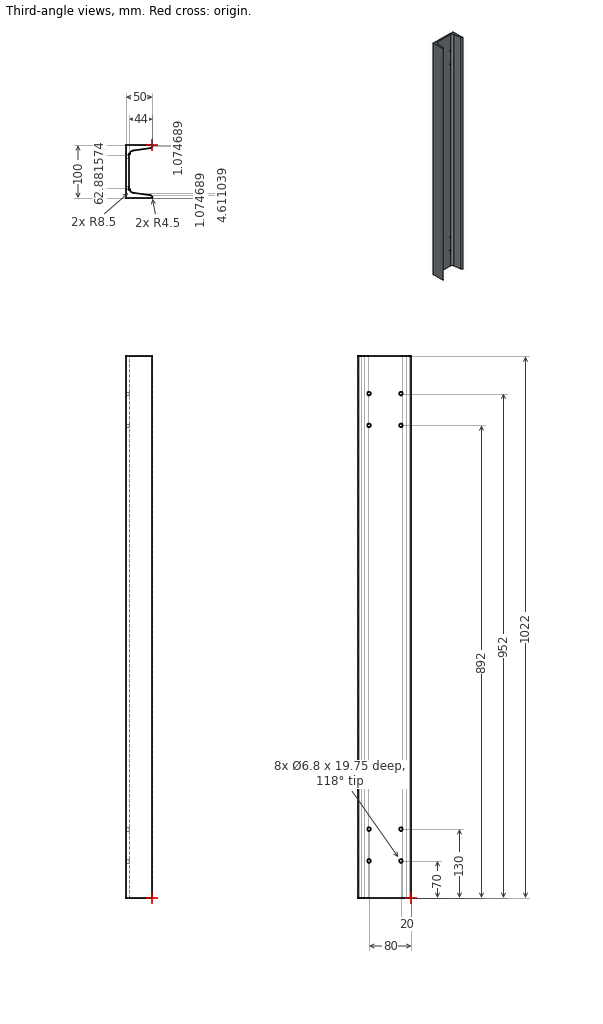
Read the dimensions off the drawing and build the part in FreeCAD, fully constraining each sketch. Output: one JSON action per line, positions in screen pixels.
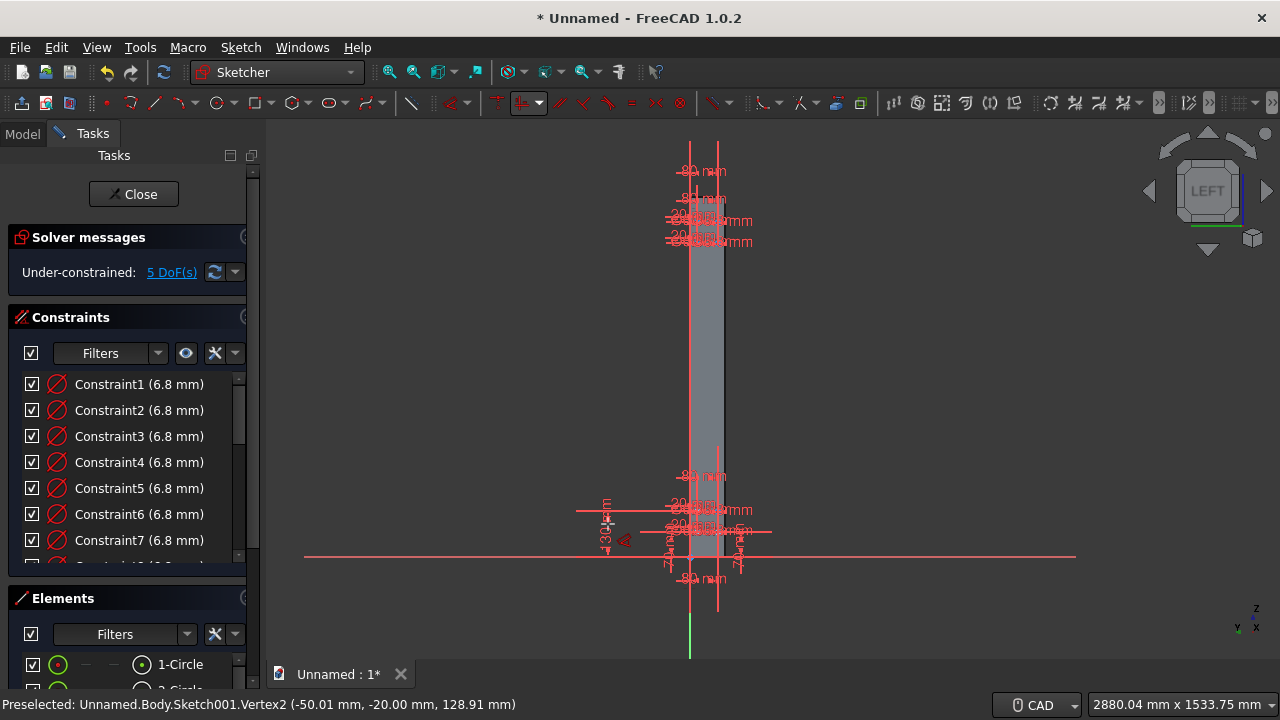
{"action": "left_click", "coordinate": [718, 512]}
{"action": "left_click", "coordinate": [776, 524]}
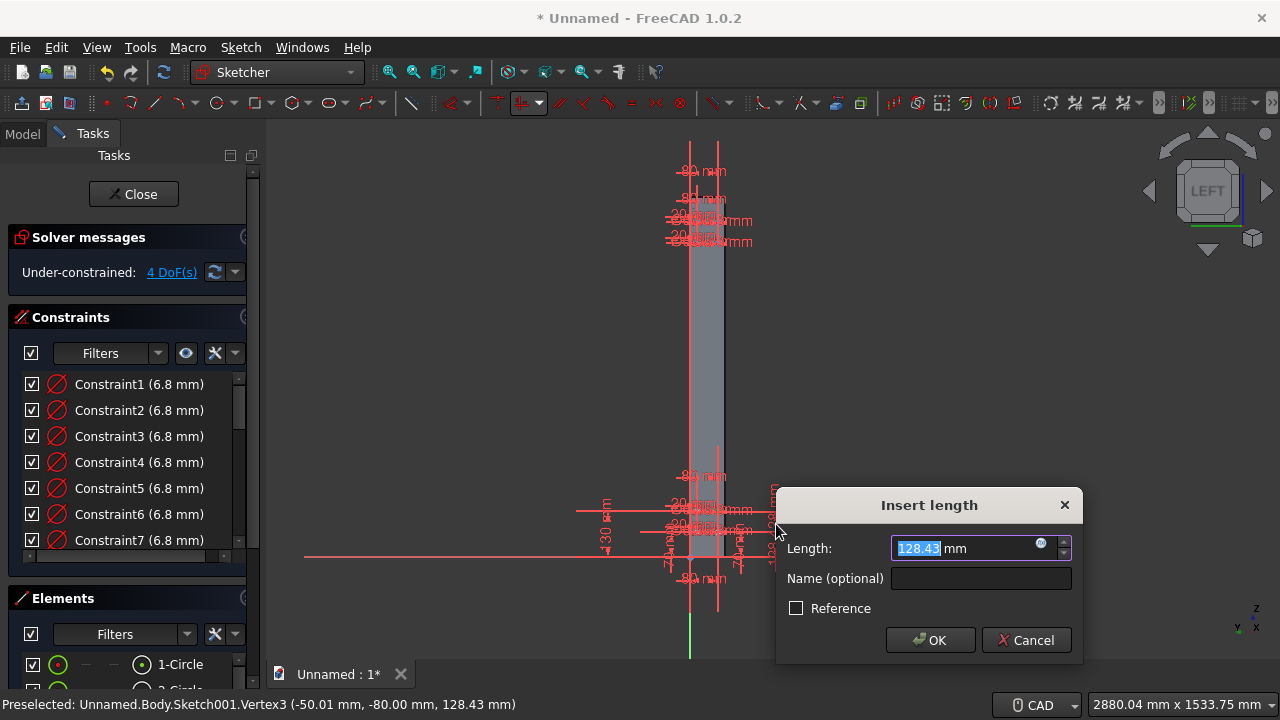
{"action": "type", "text": "130"}
{"action": "key", "text": "Return"}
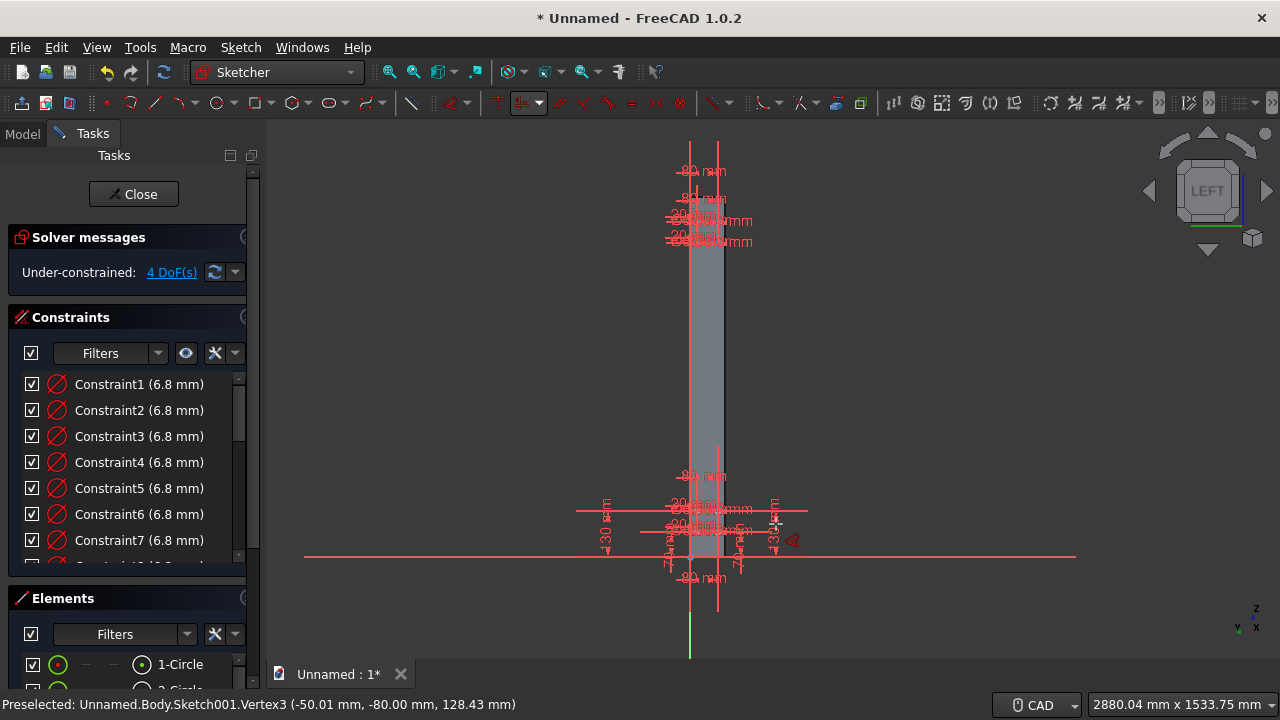
{"action": "left_click", "coordinate": [697, 243]}
{"action": "left_click", "coordinate": [656, 400]}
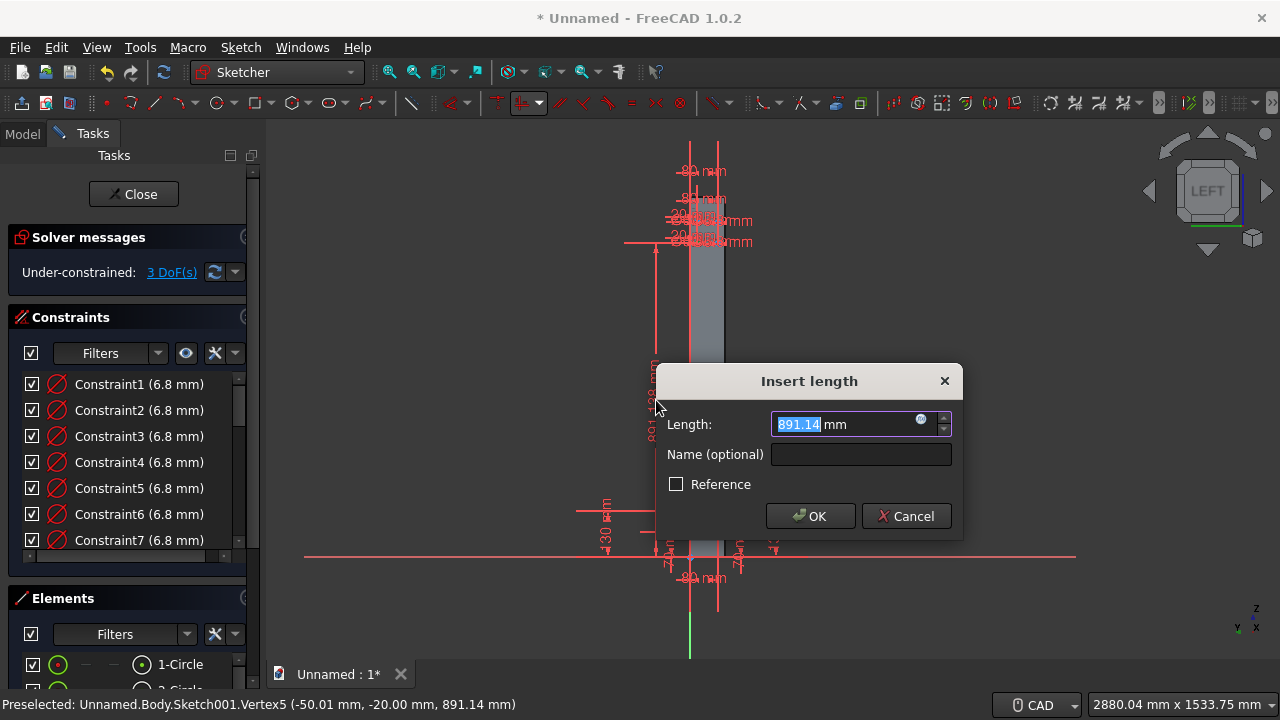
{"action": "type", "text": "892"}
{"action": "key", "text": "Return"}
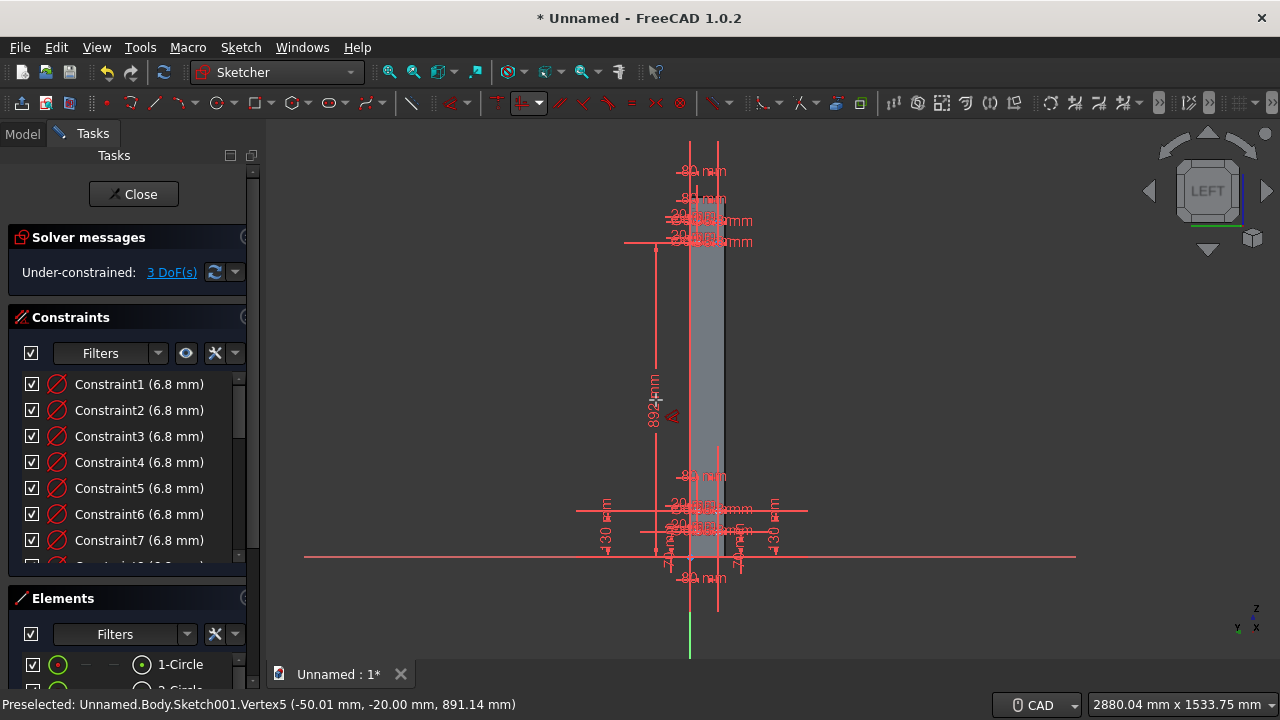
{"action": "left_click", "coordinate": [697, 222]}
{"action": "left_click", "coordinate": [656, 313]}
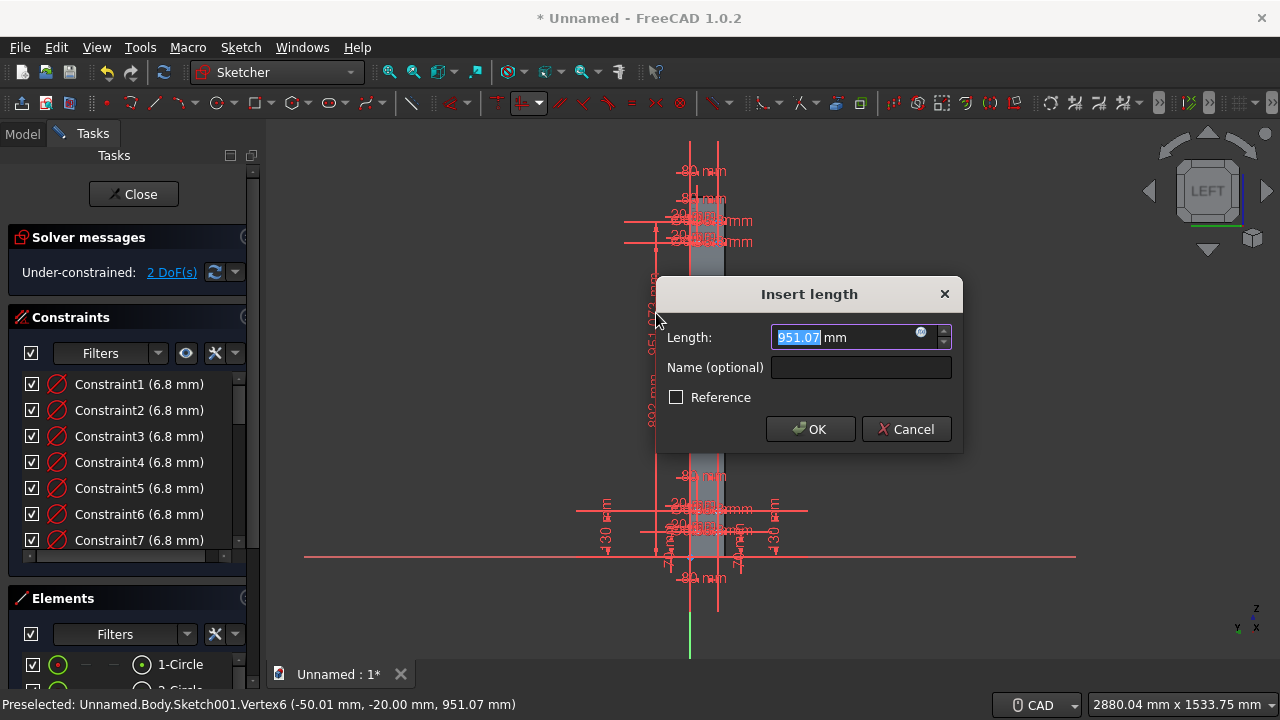
{"action": "type", "text": "952"}
{"action": "key", "text": "Return"}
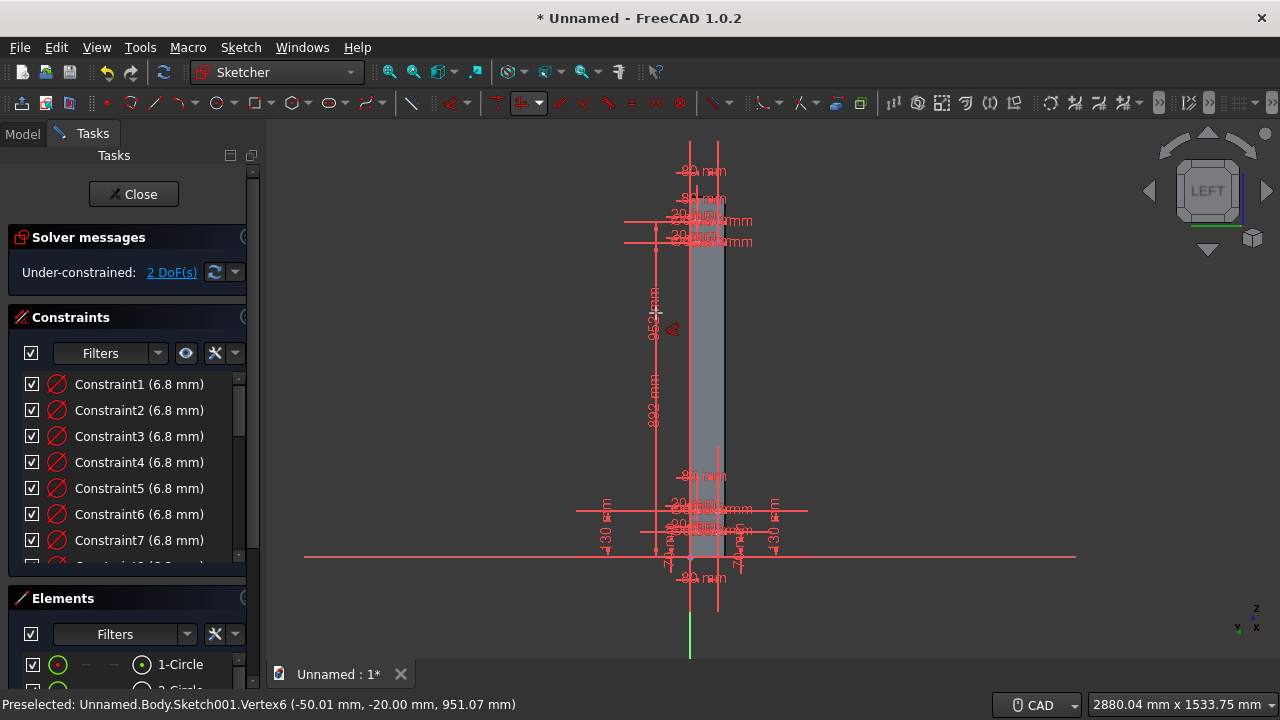
{"action": "left_click", "coordinate": [718, 223]}
{"action": "left_click", "coordinate": [656, 273]}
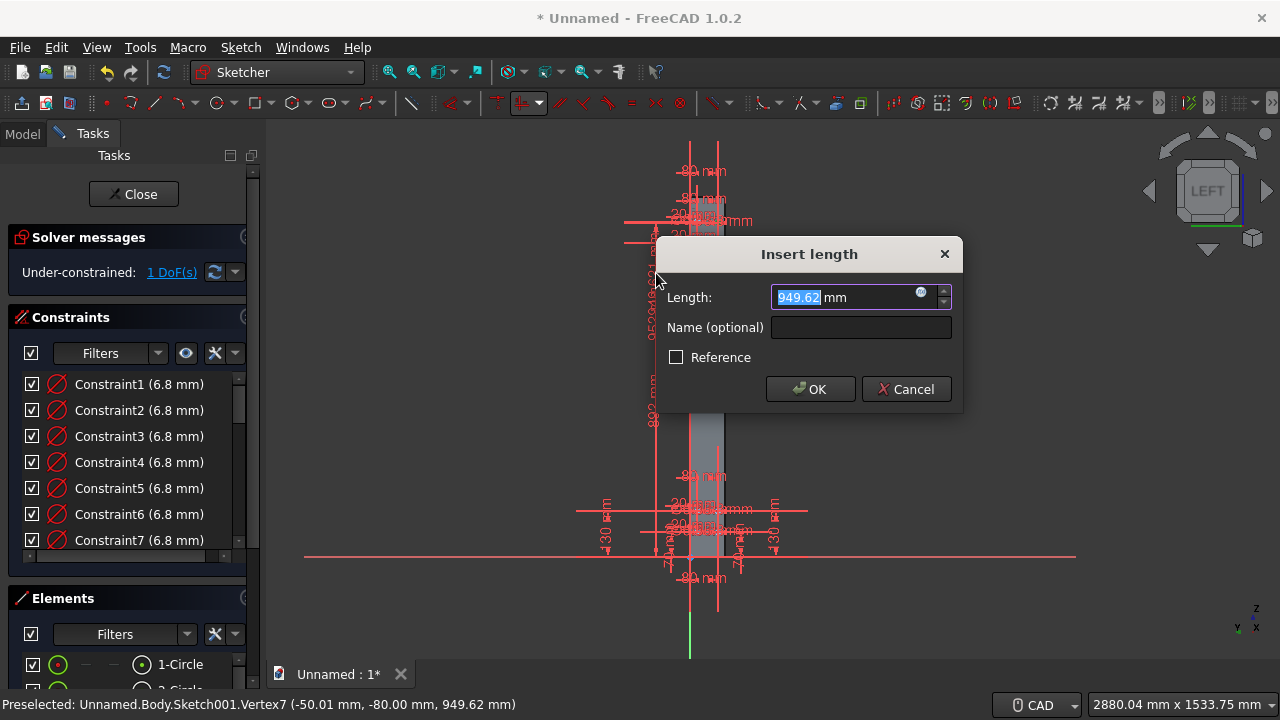
{"action": "type", "text": "952"}
{"action": "key", "text": "Return"}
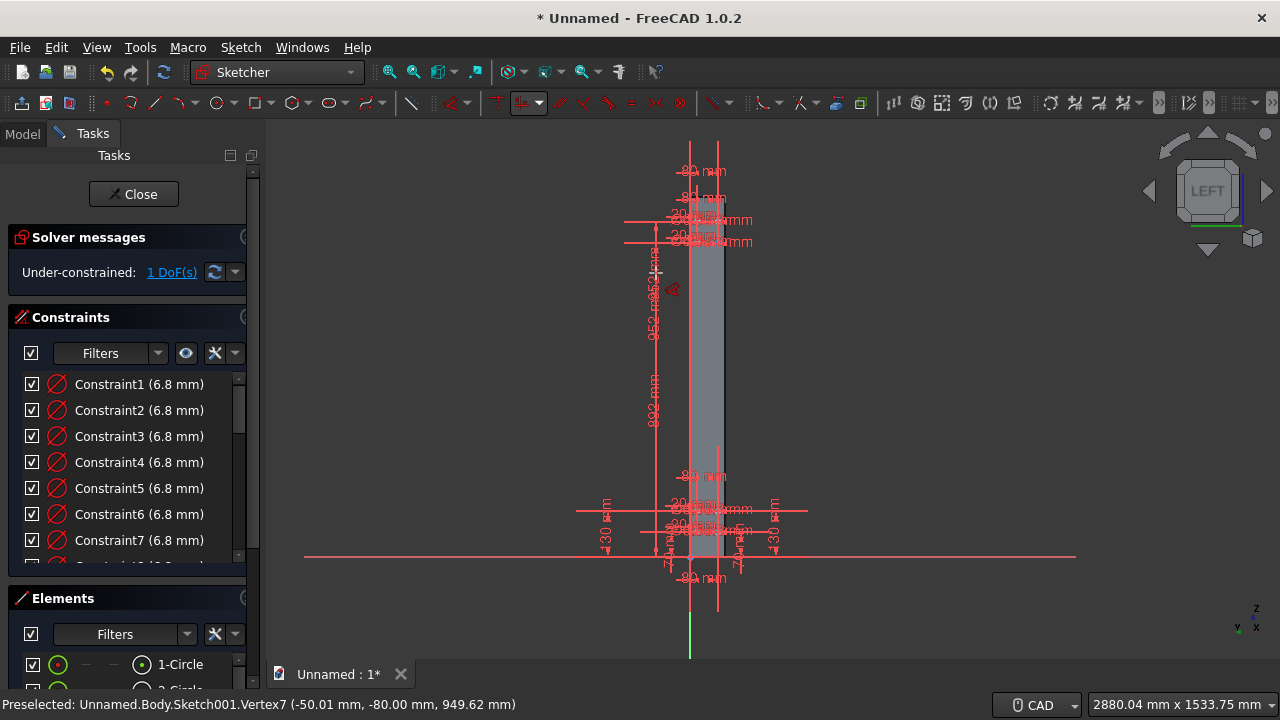
{"action": "left_click", "coordinate": [718, 244]}
{"action": "left_click", "coordinate": [752, 400]}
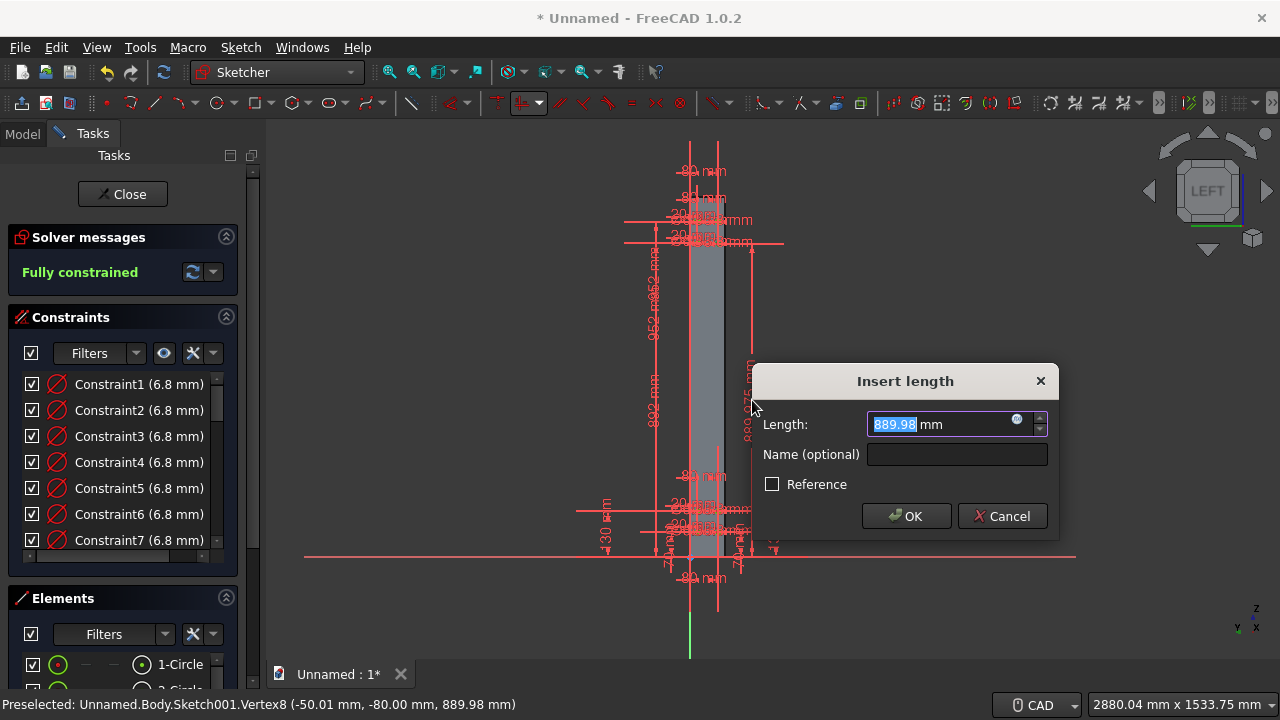
{"action": "type", "text": "892"}
{"action": "key", "text": "Return"}
{"action": "key", "text": "Escape"}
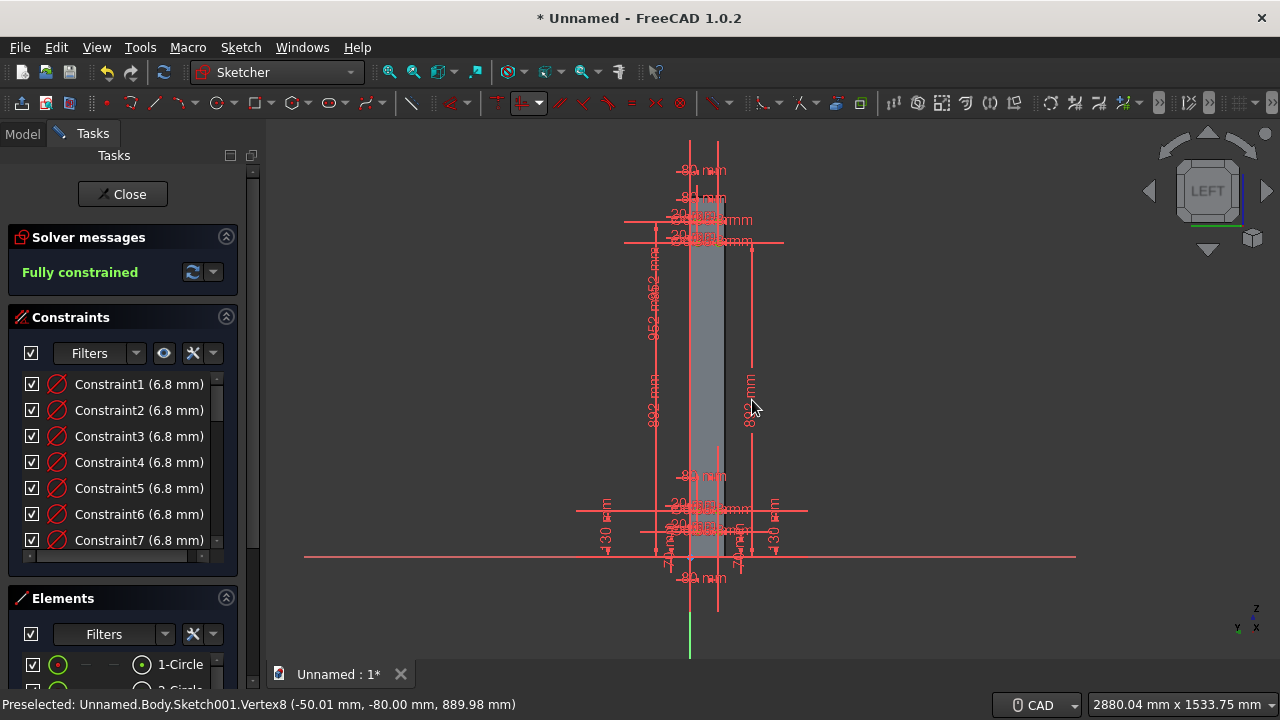
{"action": "left_click", "coordinate": [123, 194]}